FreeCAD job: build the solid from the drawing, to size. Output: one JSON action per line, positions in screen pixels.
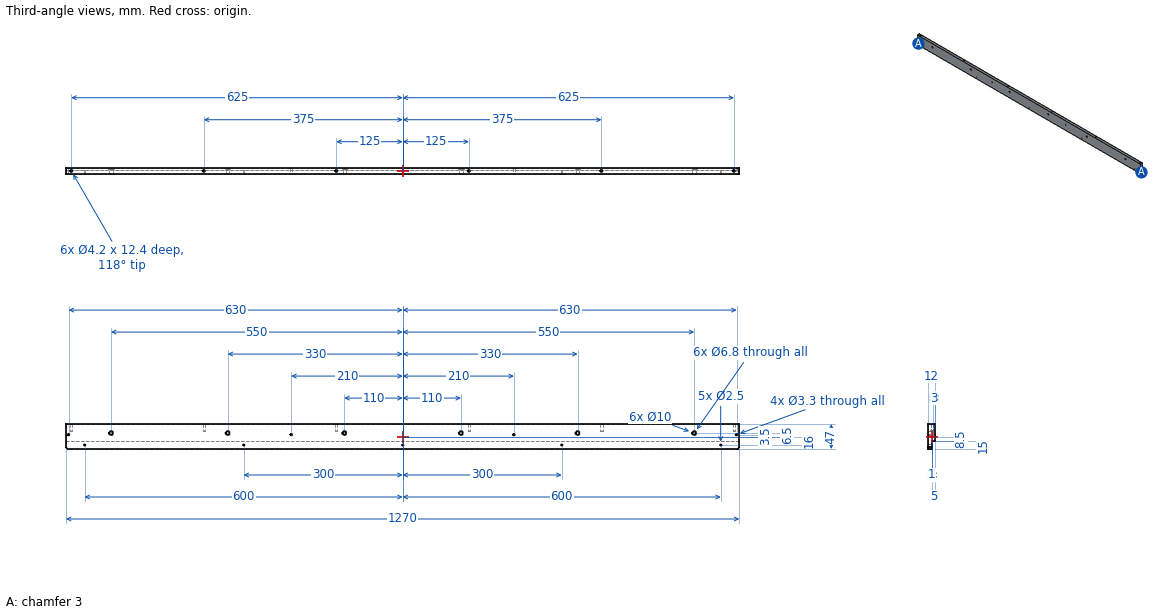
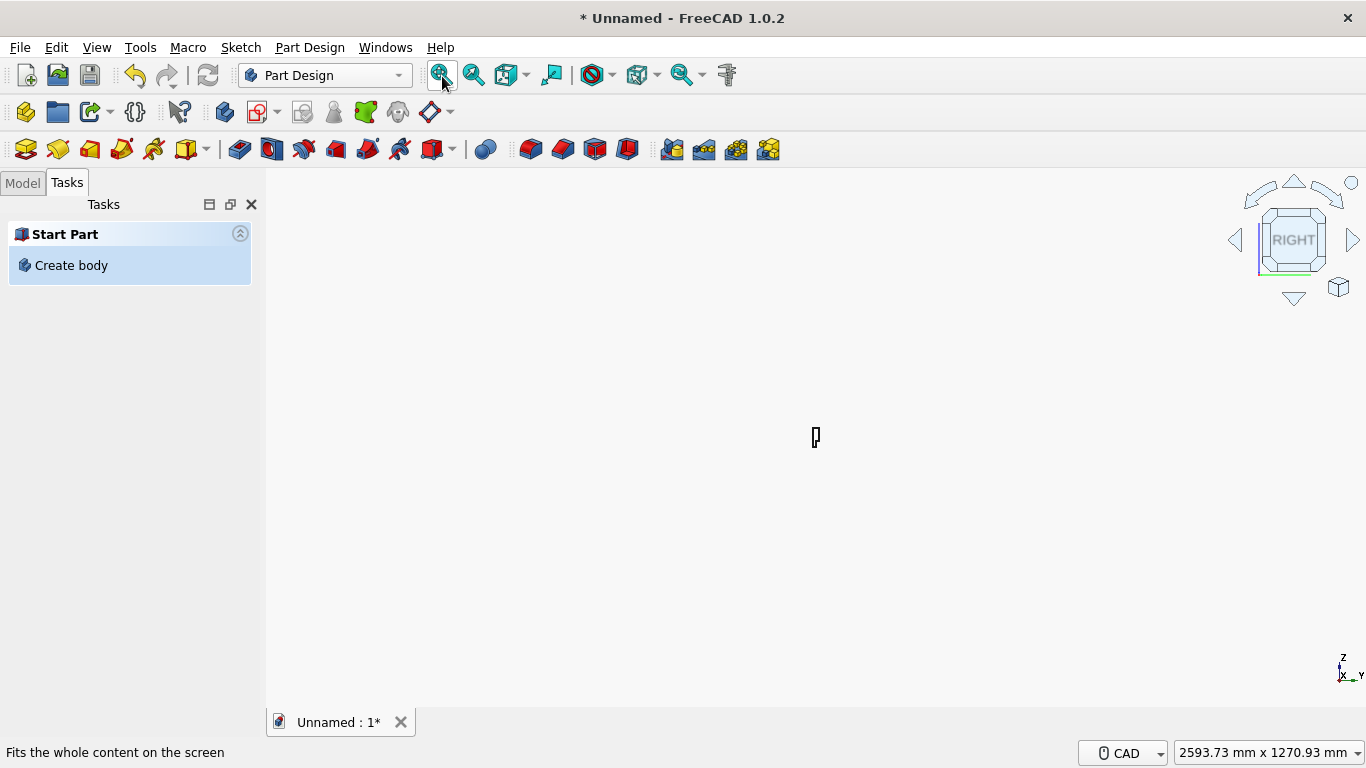
{"action": "scroll", "coordinate": [815, 446], "scroll_direction": "up", "scroll_amount": 14}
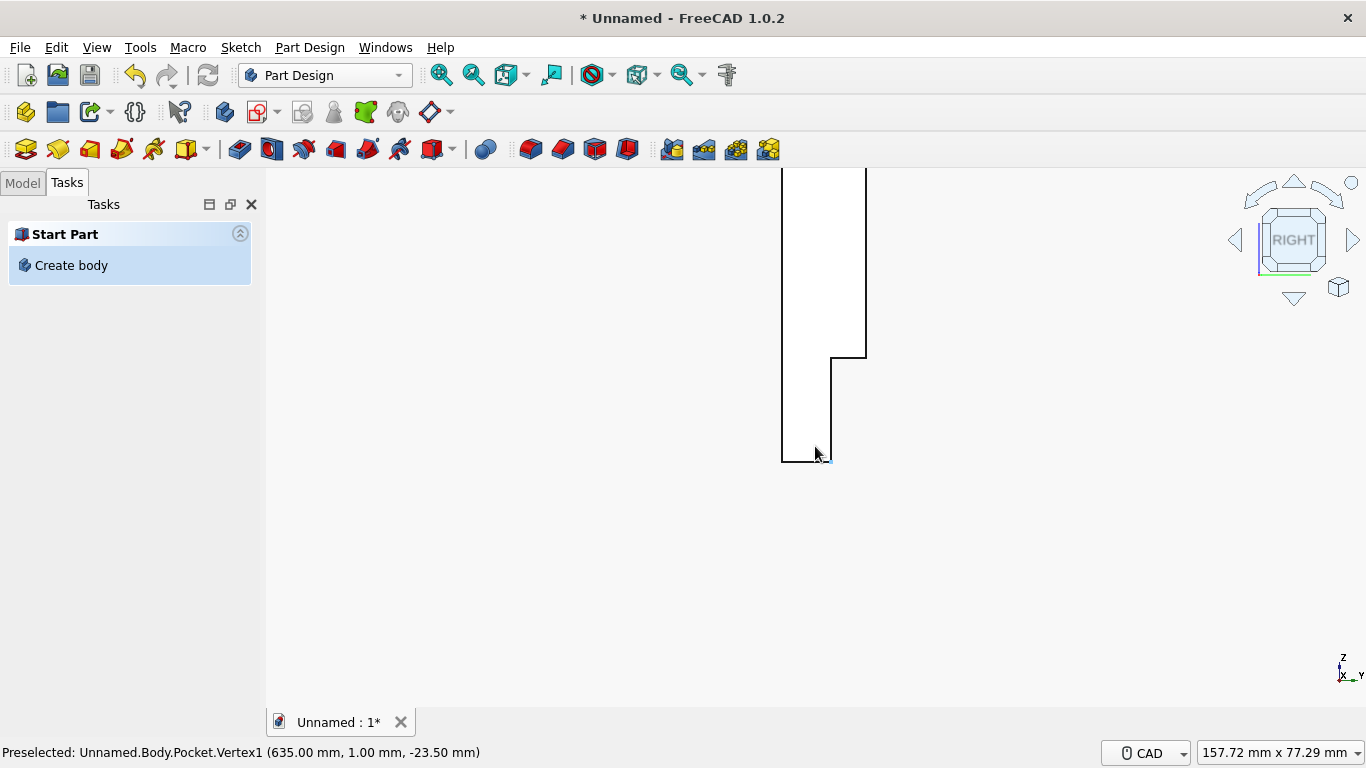
{"action": "left_click", "coordinate": [806, 461]}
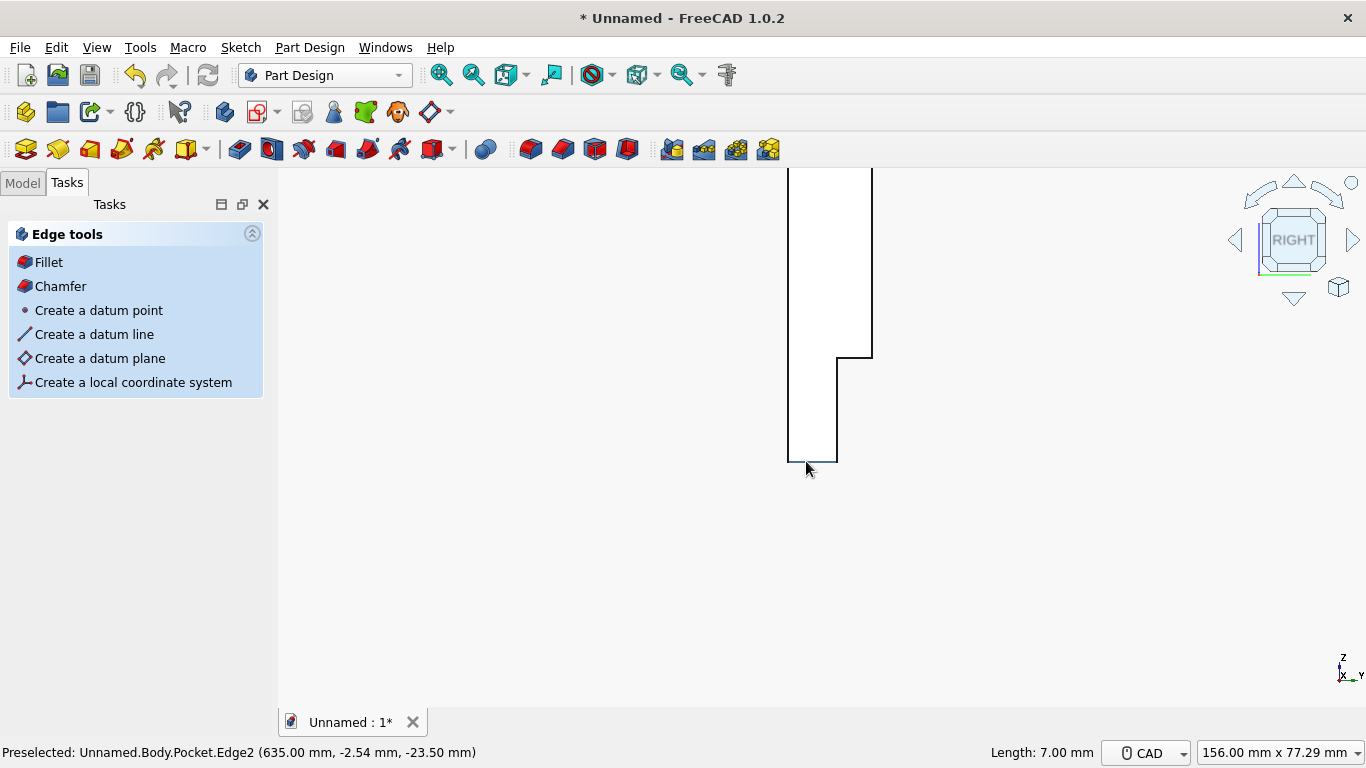
{"action": "key", "text": "v f"}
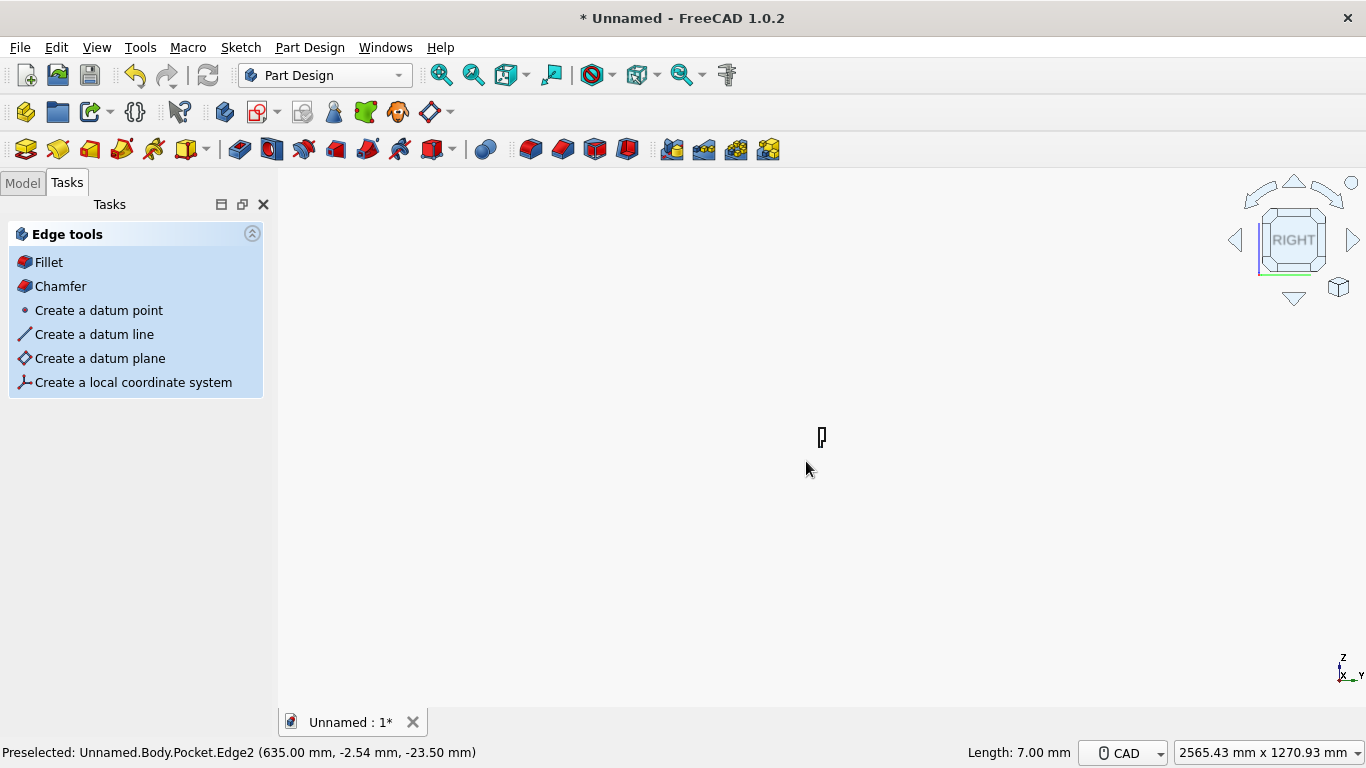
{"action": "key", "text": "5"}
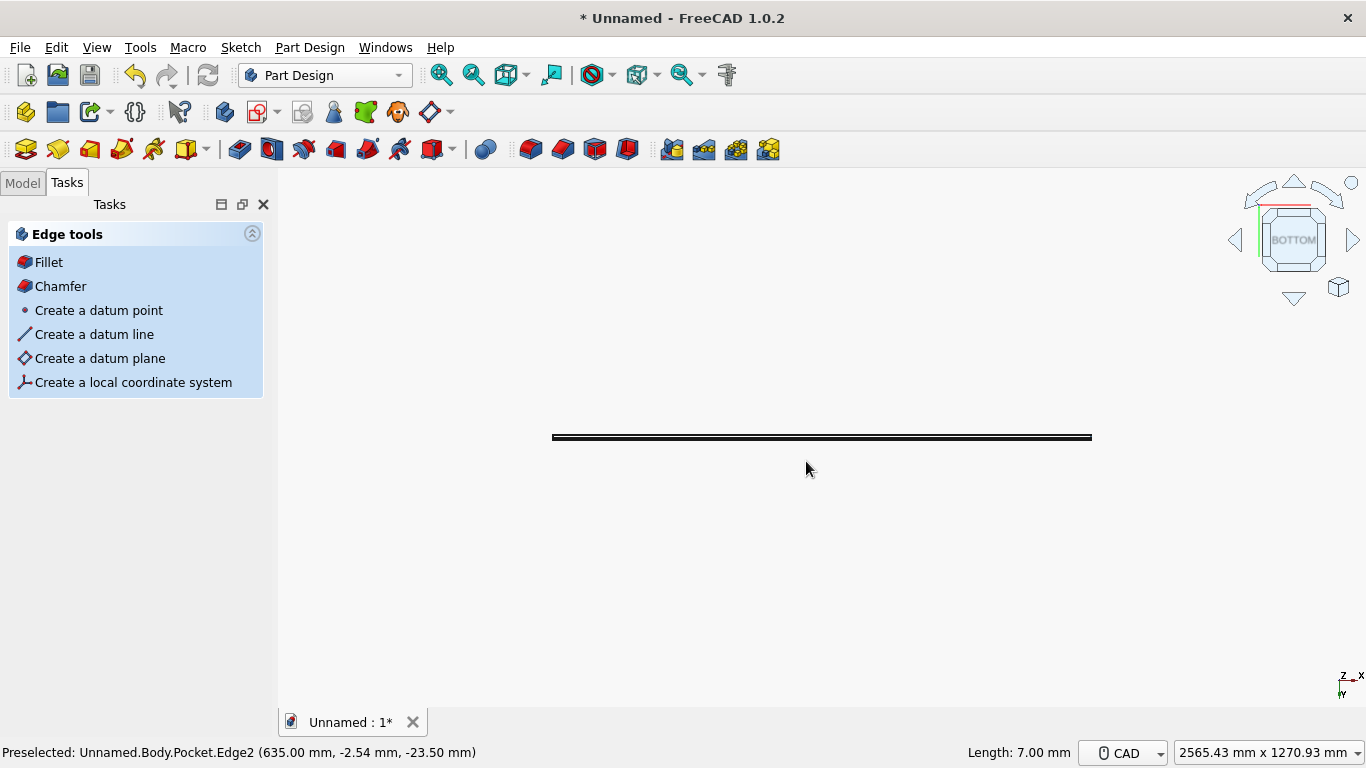
{"action": "scroll", "coordinate": [553, 435], "scroll_direction": "up", "scroll_amount": 14}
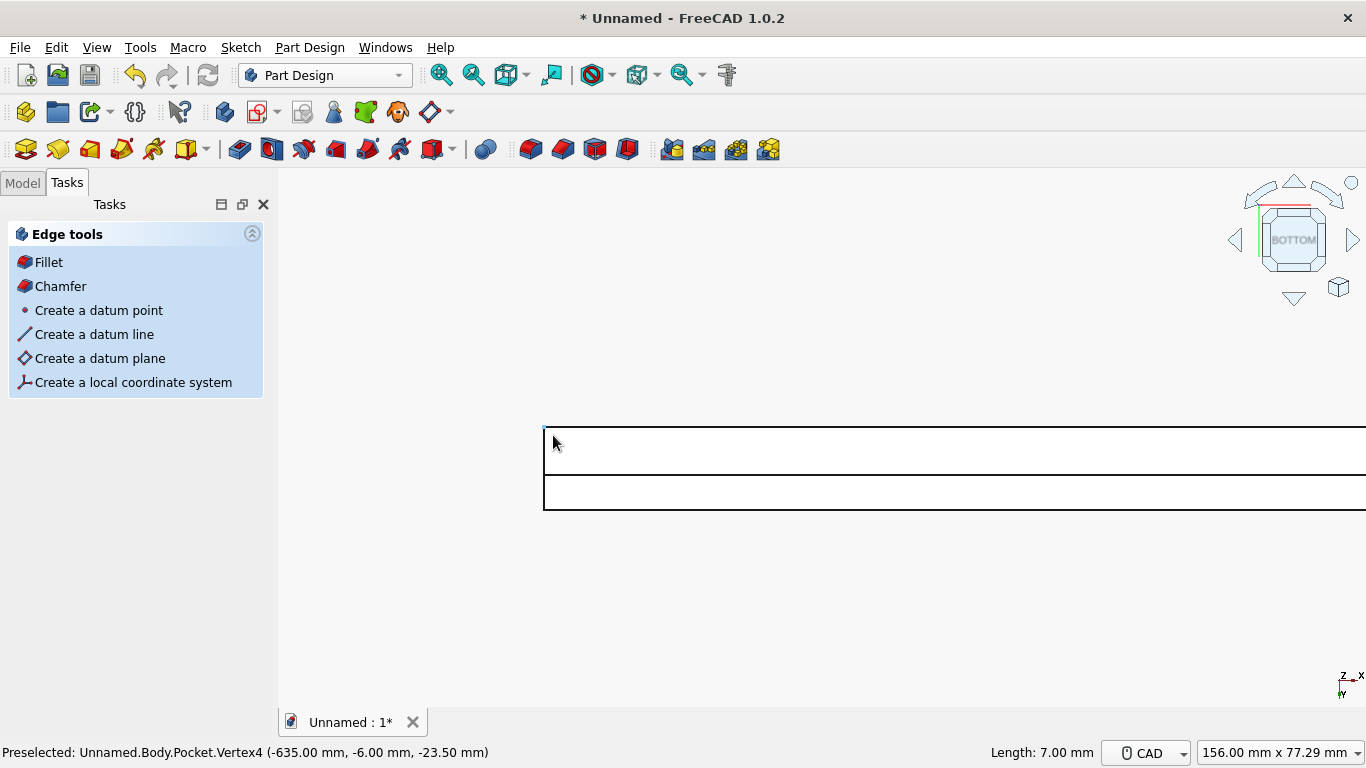
{"action": "left_click", "coordinate": [544, 450], "text": "ctrl"}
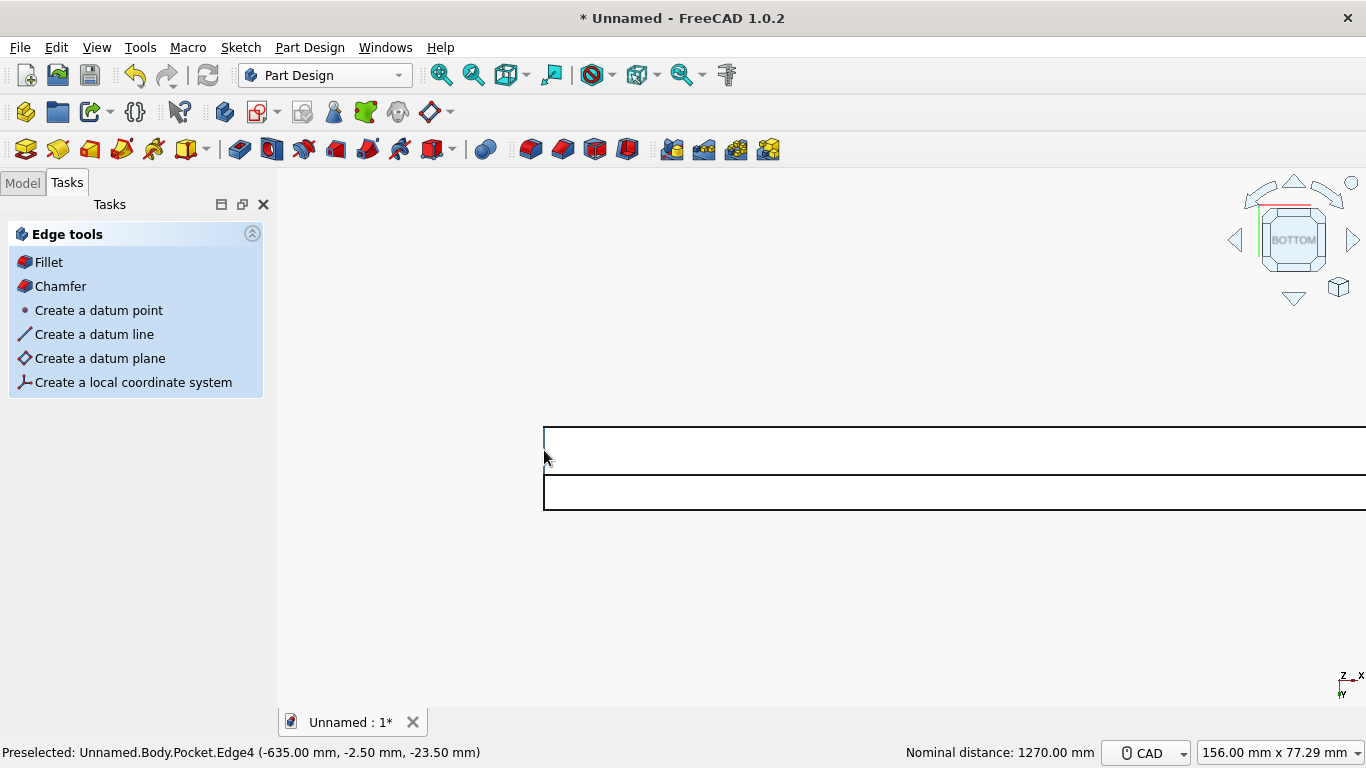
{"action": "left_click", "coordinate": [564, 150]}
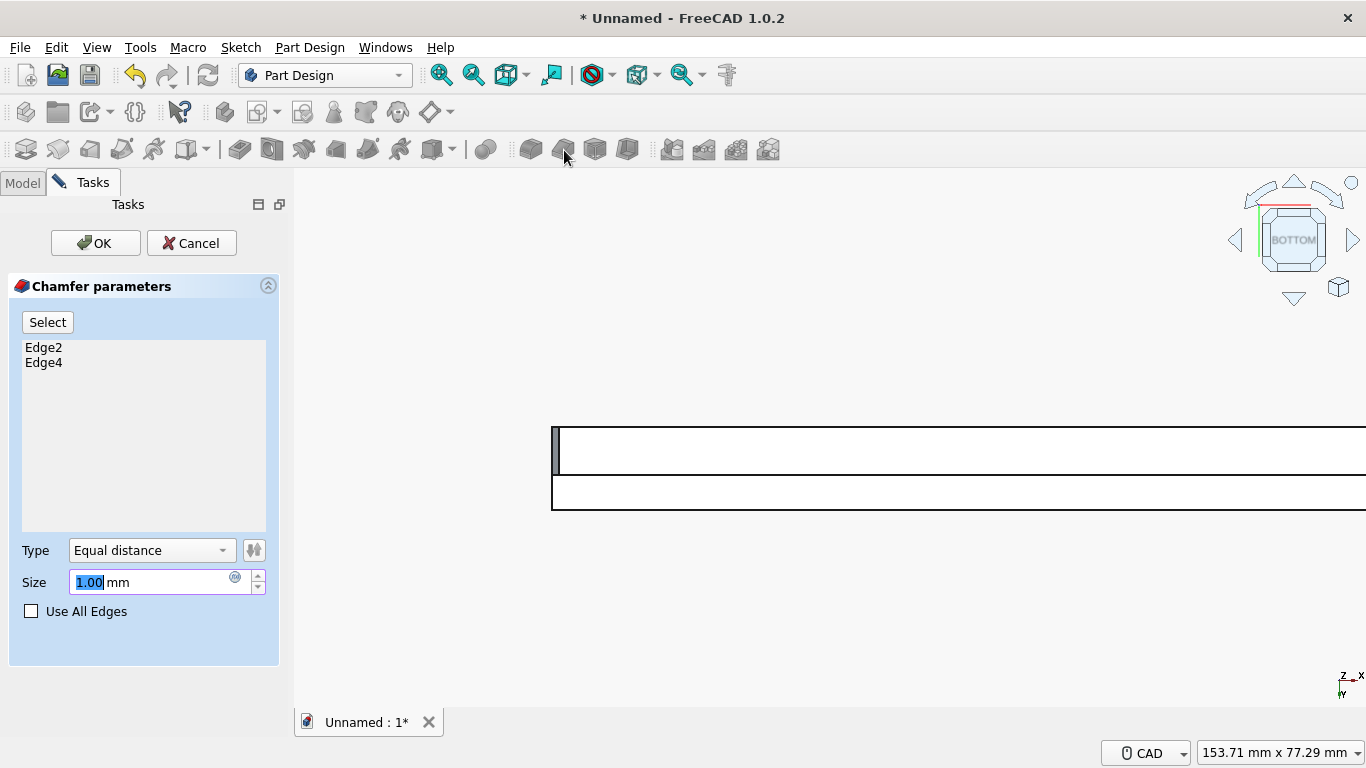
{"action": "type", "text": "3"}
{"action": "key", "text": "Tab"}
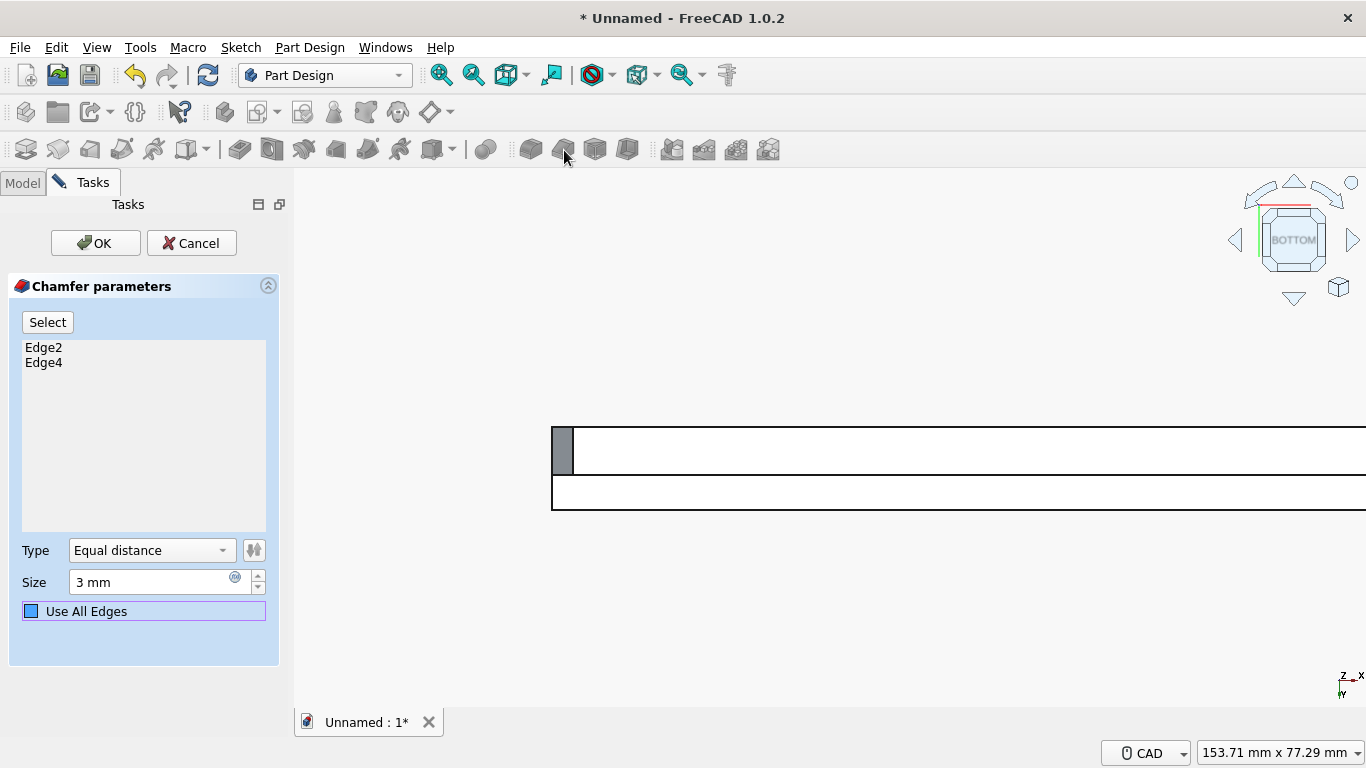
{"action": "left_click", "coordinate": [96, 243]}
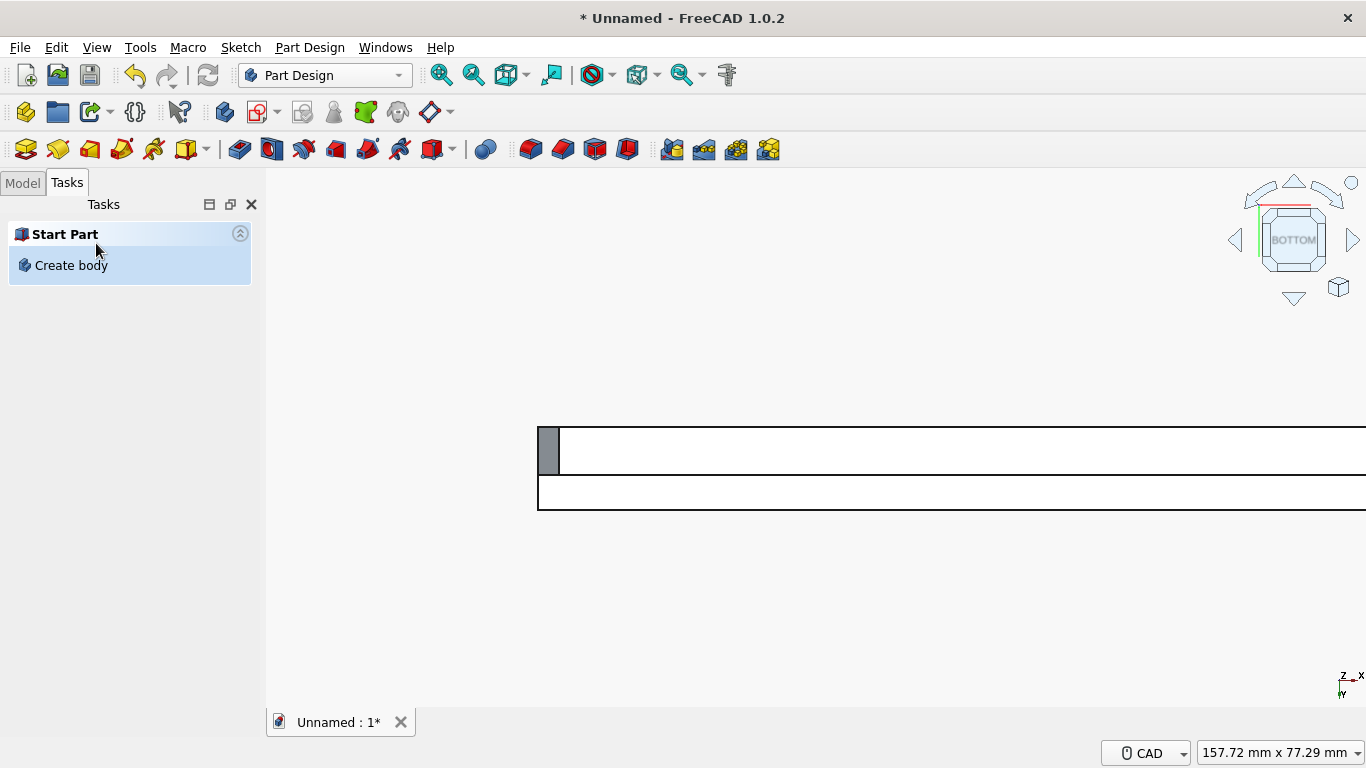
{"action": "left_click", "coordinate": [442, 76]}